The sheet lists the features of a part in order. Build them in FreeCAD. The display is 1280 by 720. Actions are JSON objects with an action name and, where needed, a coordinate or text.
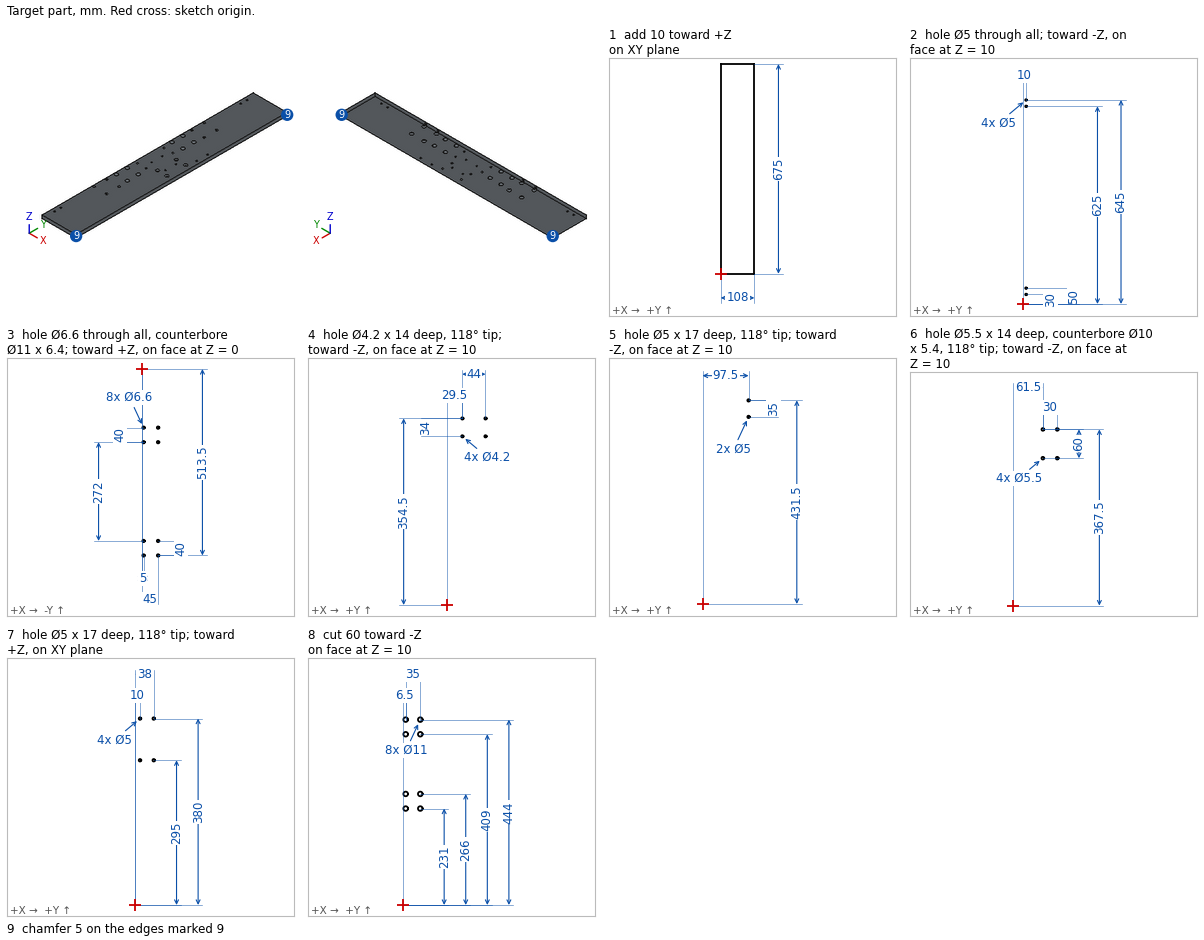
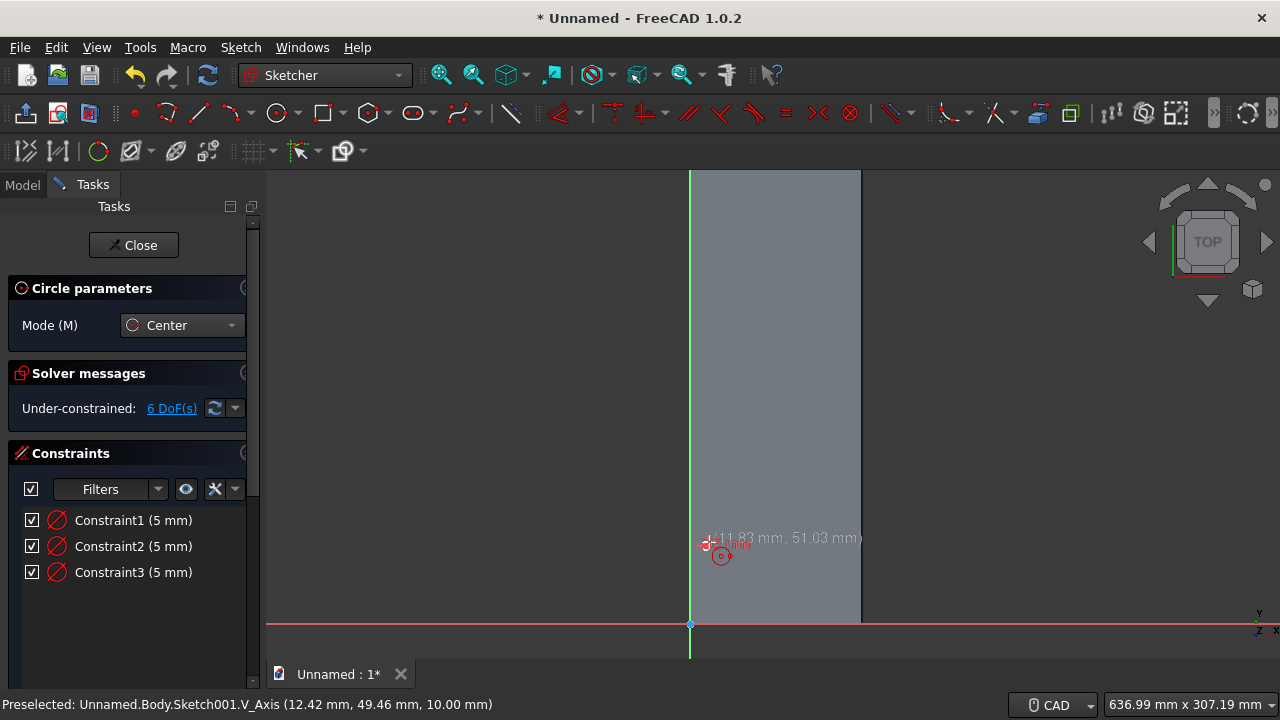
{"action": "scroll", "coordinate": [706, 576], "scroll_direction": "up", "scroll_amount": 9}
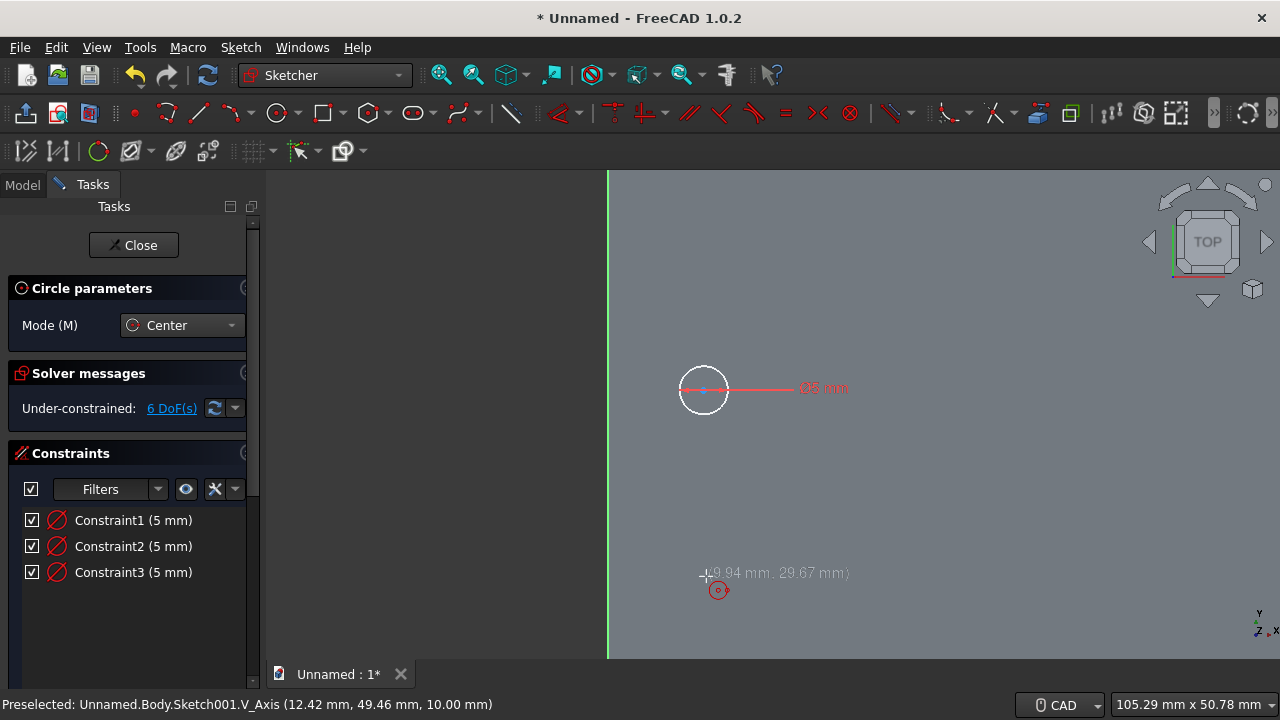
{"action": "scroll", "coordinate": [706, 554], "scroll_direction": "down", "scroll_amount": 15}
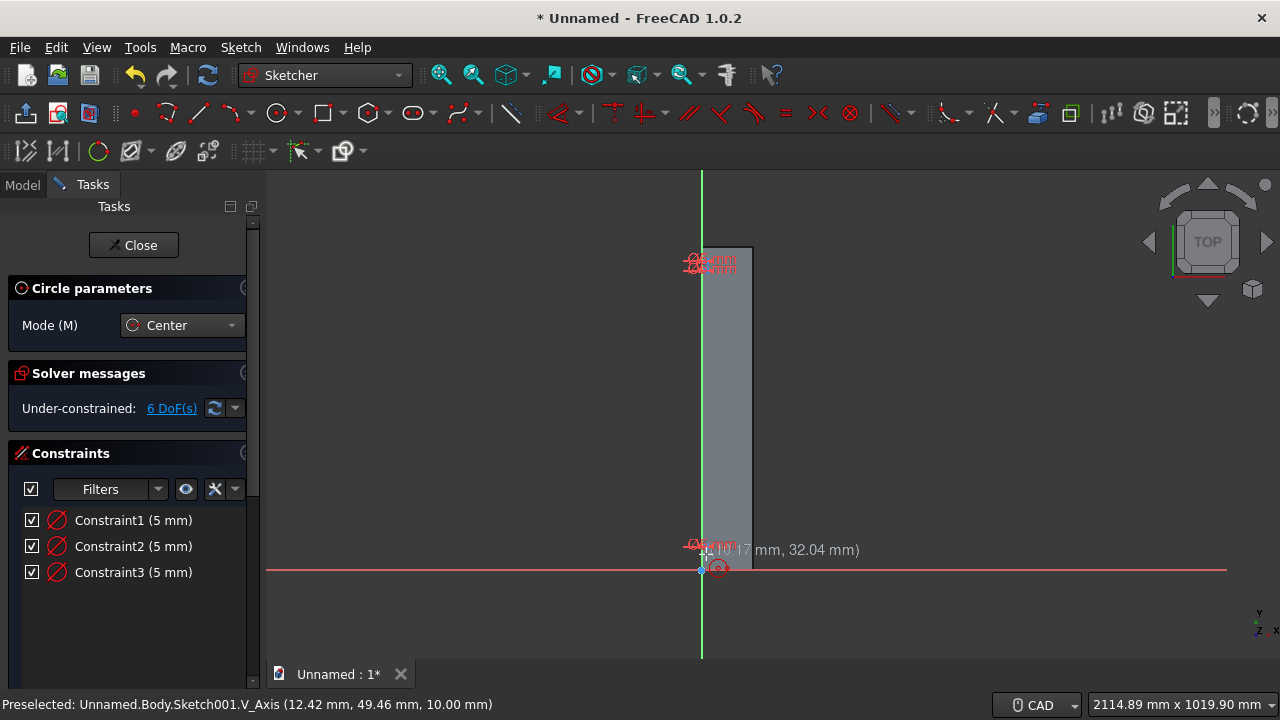
{"action": "scroll", "coordinate": [706, 556], "scroll_direction": "up", "scroll_amount": 6}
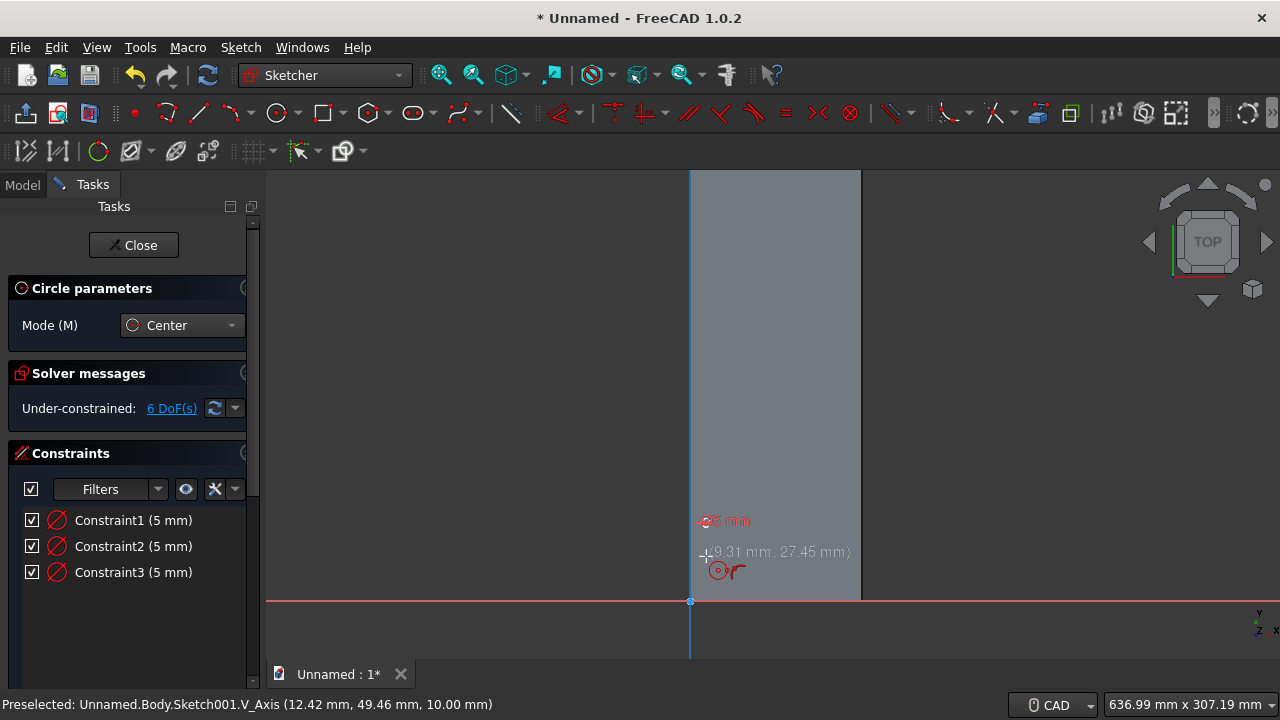
{"action": "left_click", "coordinate": [706, 553]}
{"action": "mouse_move", "coordinate": [709, 551]}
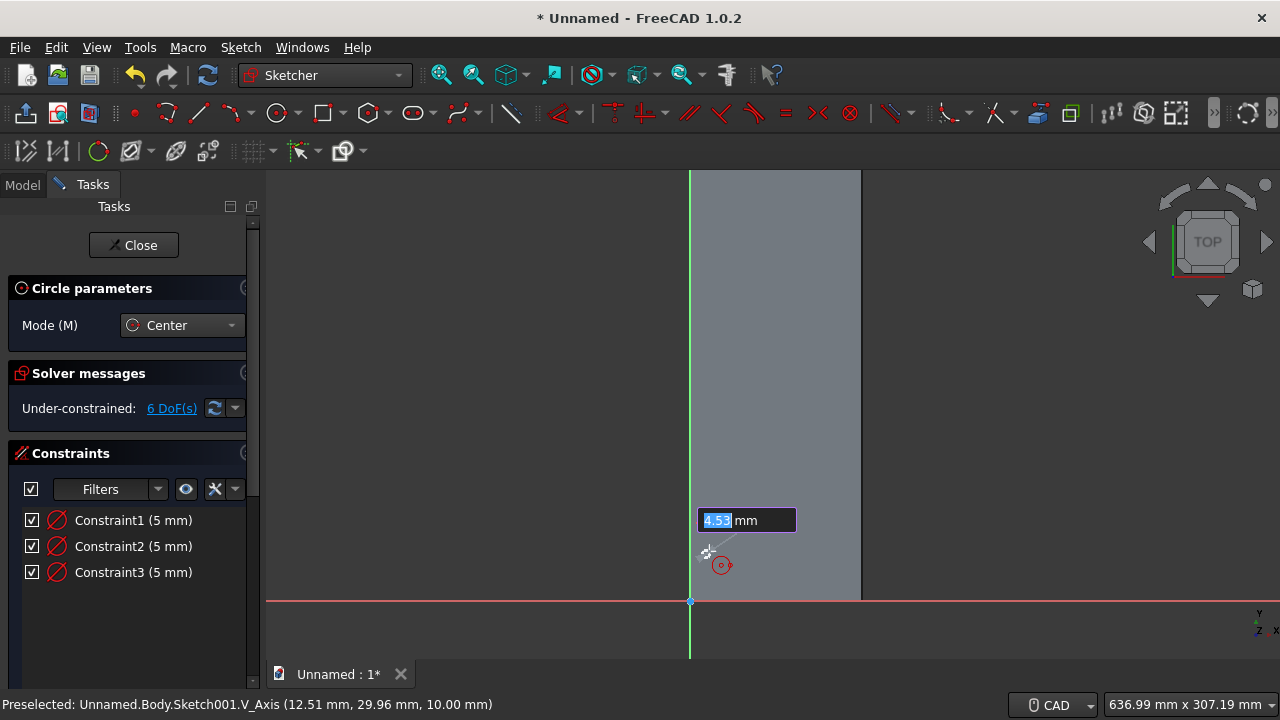
{"action": "type", "text": "5"}
{"action": "key", "text": "Return"}
{"action": "key", "text": "Escape"}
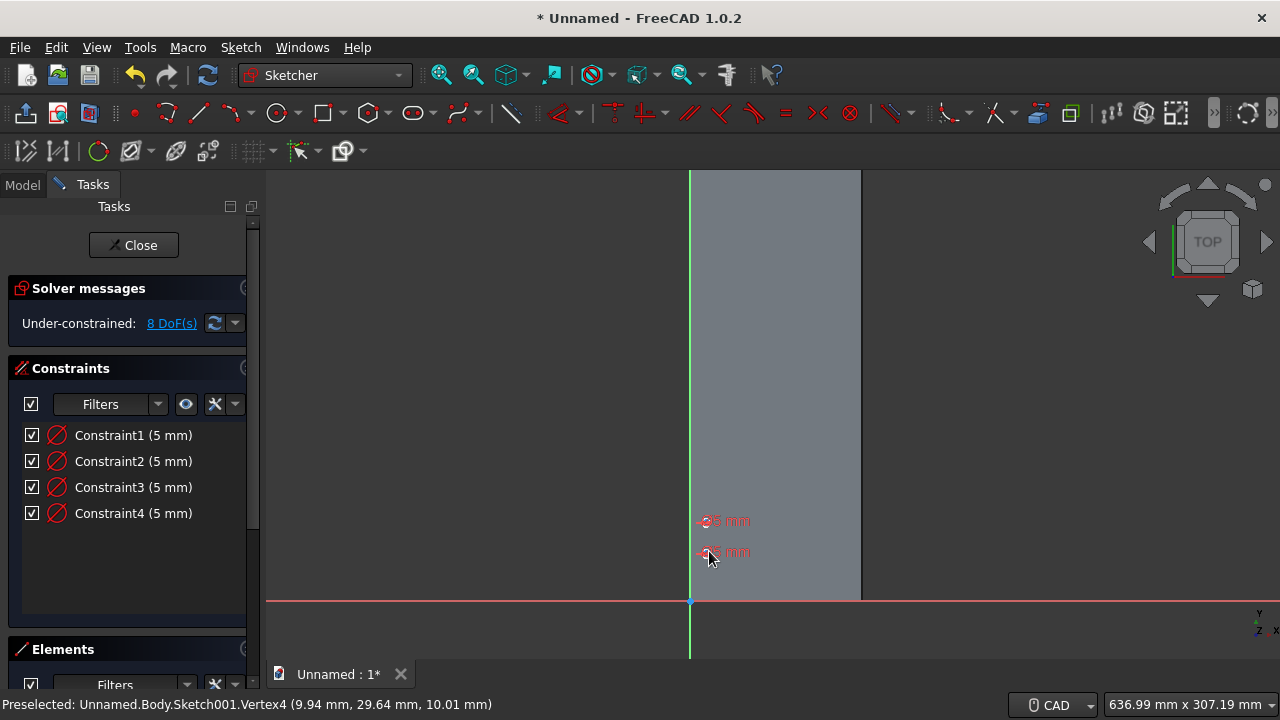
{"action": "scroll", "coordinate": [706, 556], "scroll_direction": "down", "scroll_amount": 6}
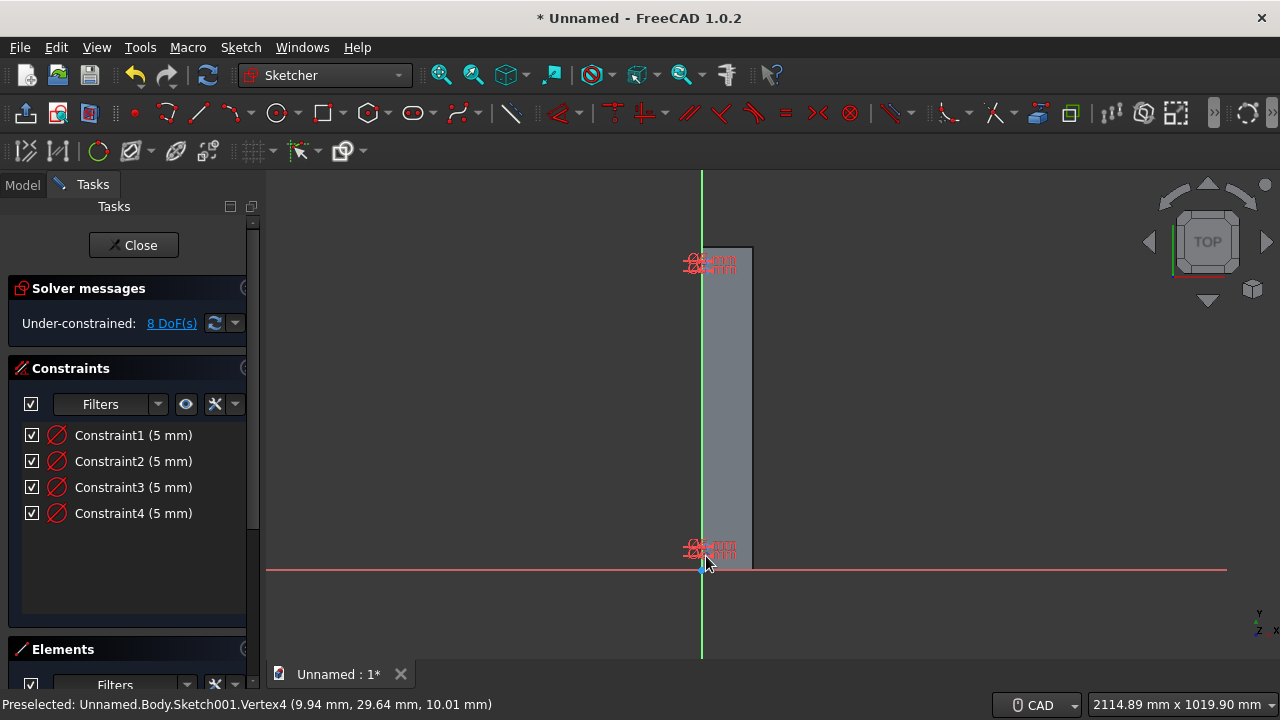
{"action": "scroll", "coordinate": [706, 261], "scroll_direction": "up", "scroll_amount": 2}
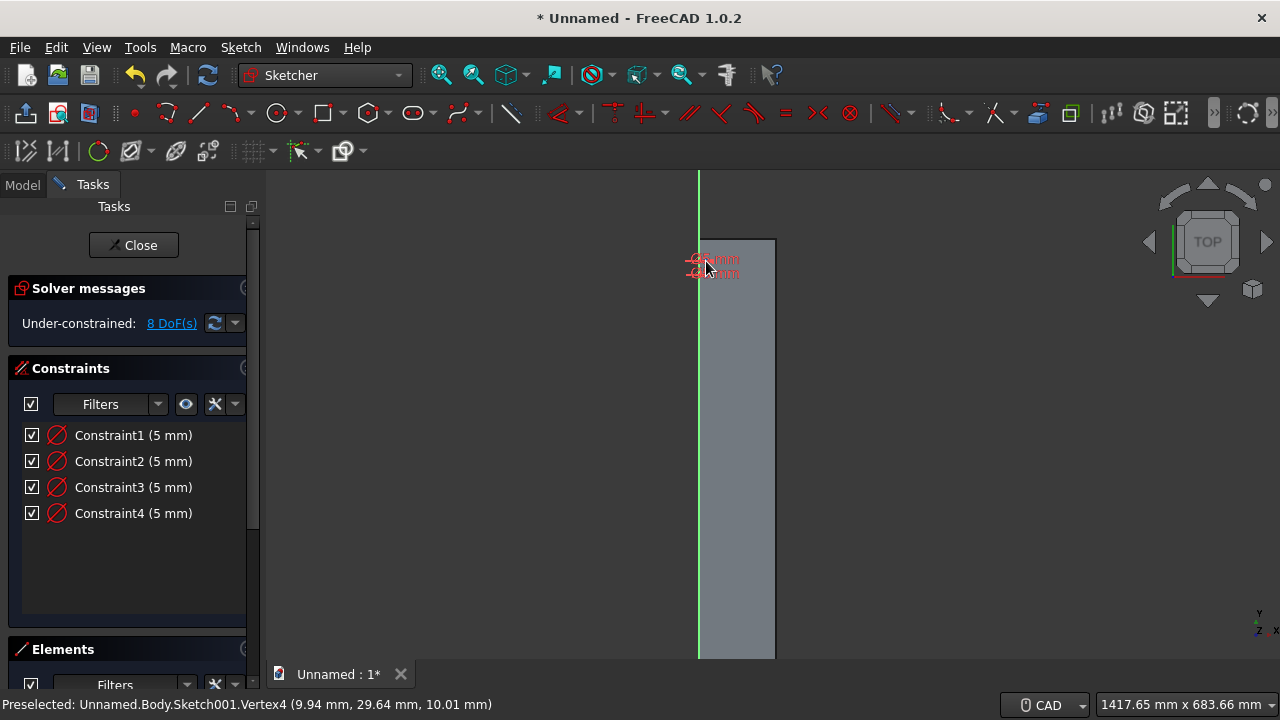
{"action": "left_click", "coordinate": [706, 261]}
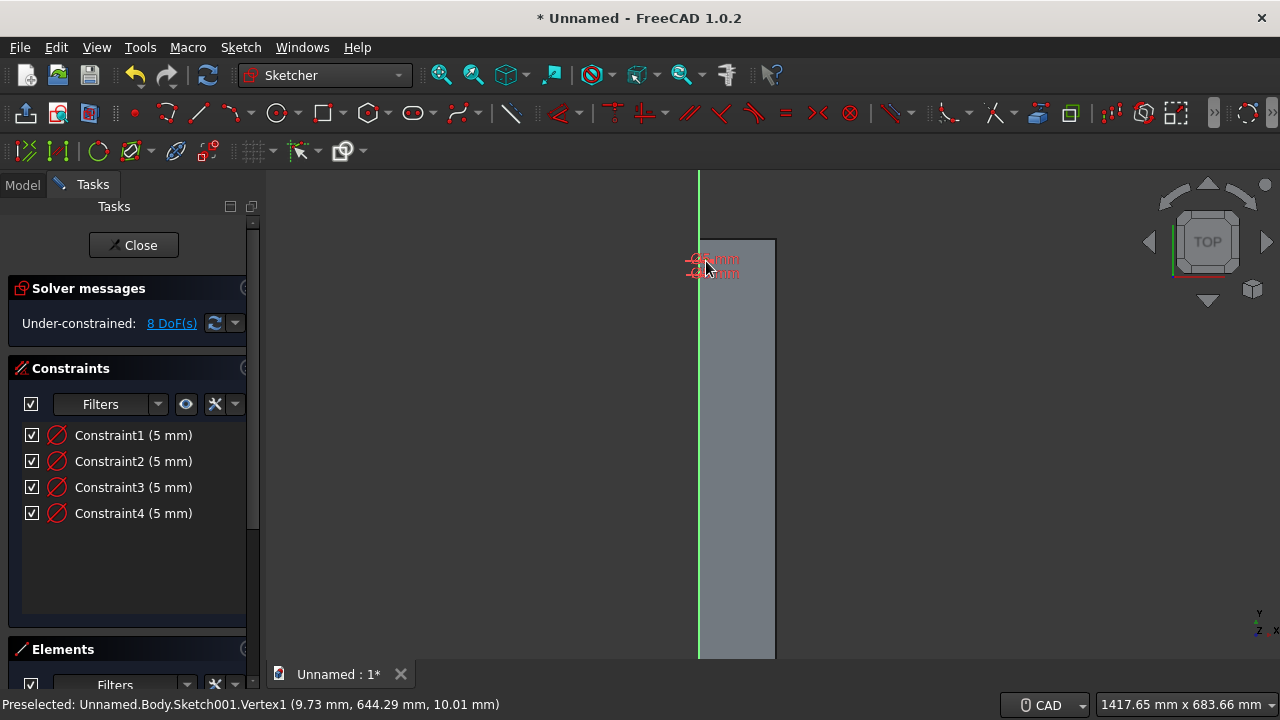
{"action": "left_click", "coordinate": [706, 275]}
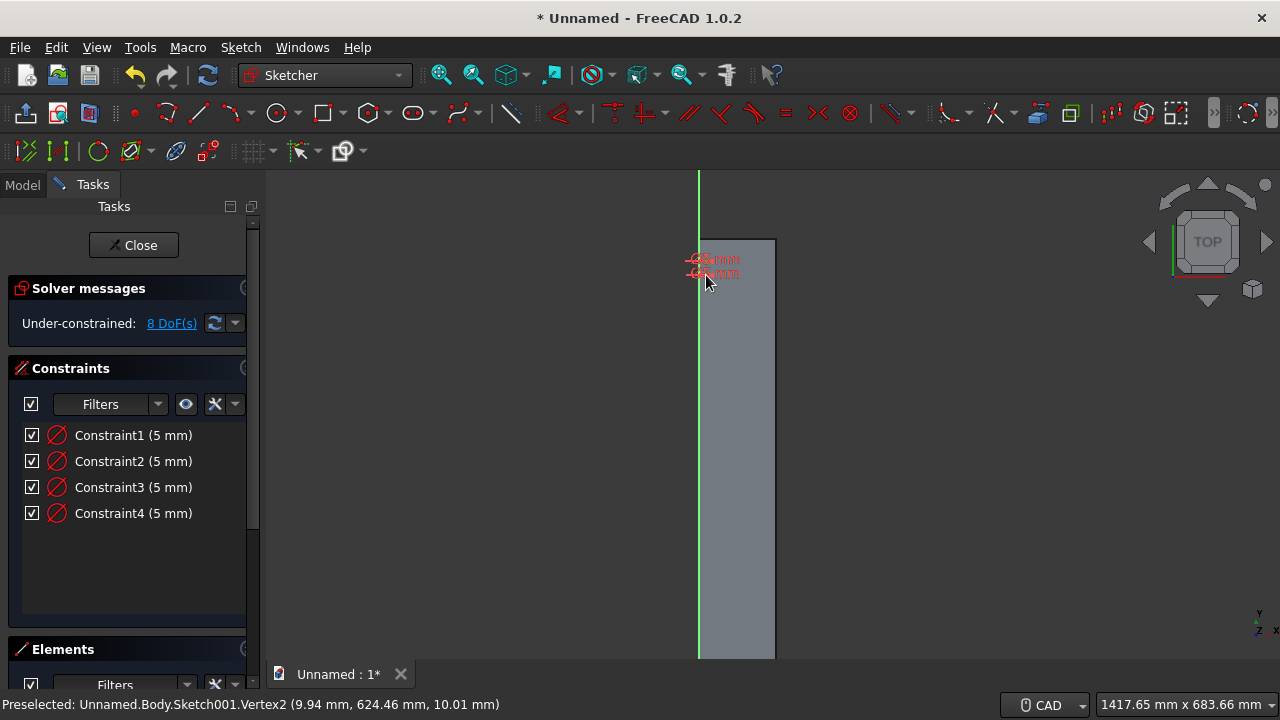
{"action": "left_click", "coordinate": [668, 114]}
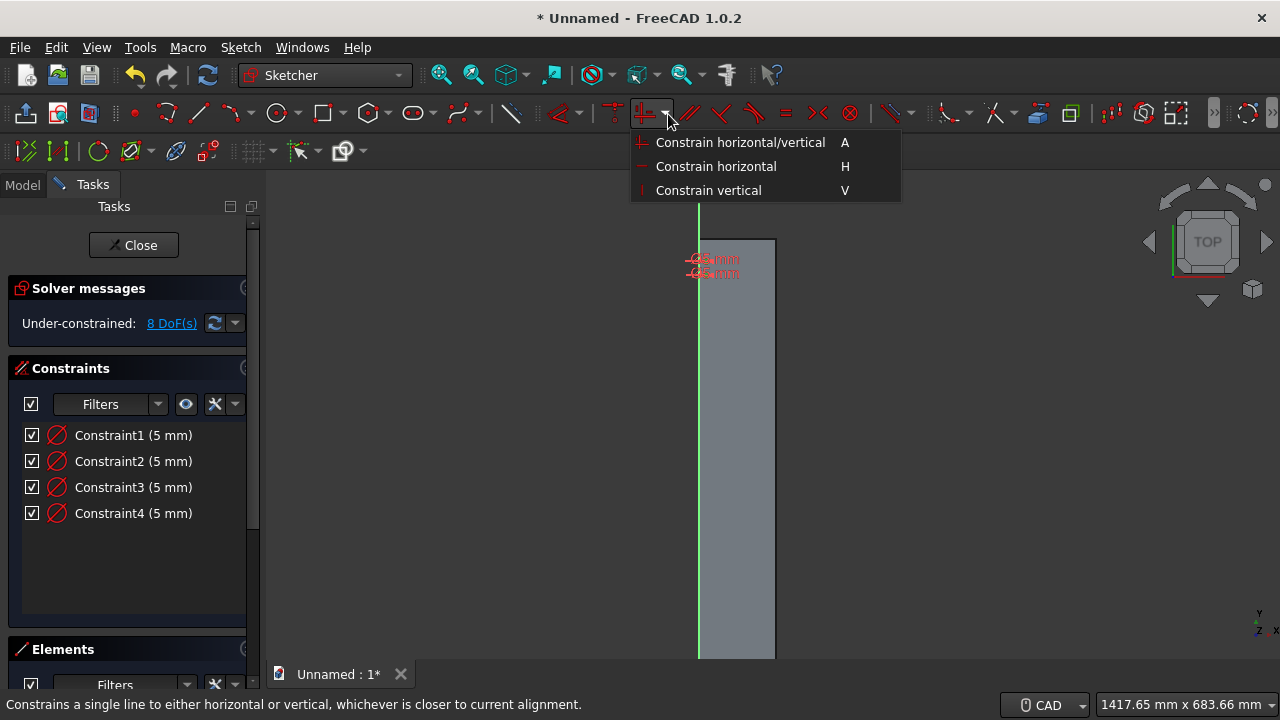
{"action": "left_click", "coordinate": [766, 190]}